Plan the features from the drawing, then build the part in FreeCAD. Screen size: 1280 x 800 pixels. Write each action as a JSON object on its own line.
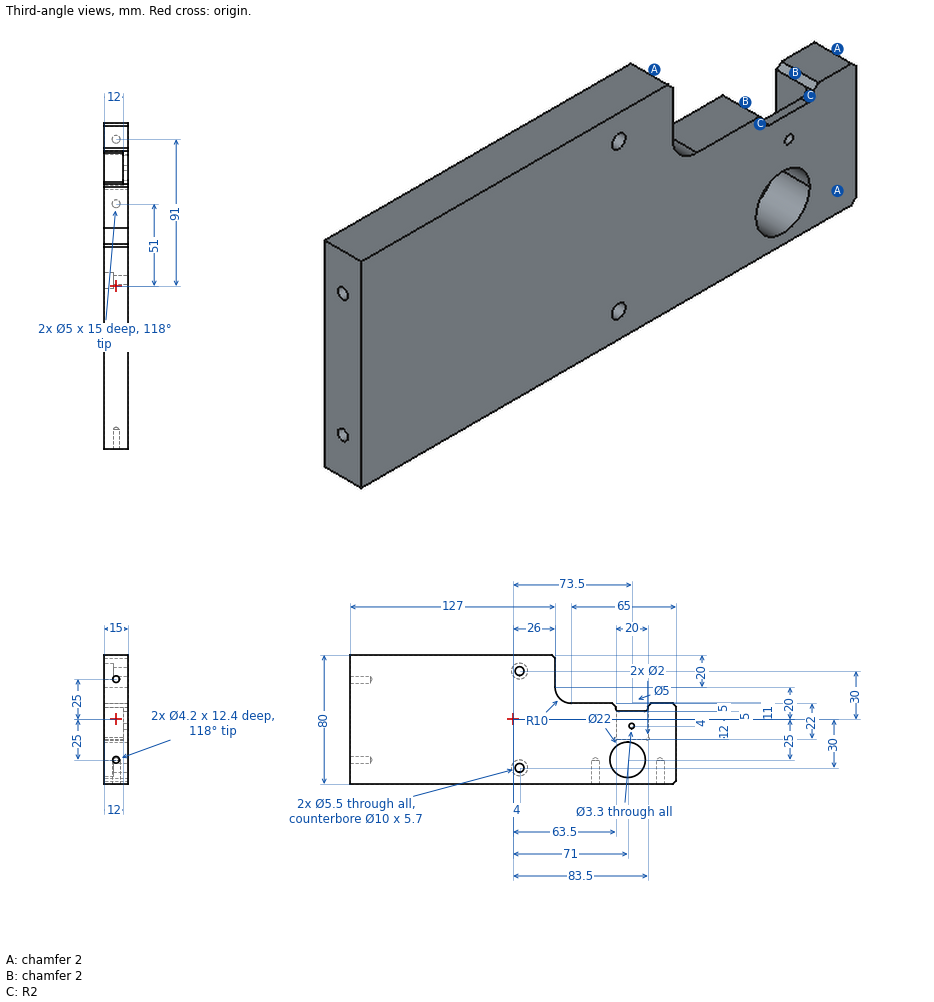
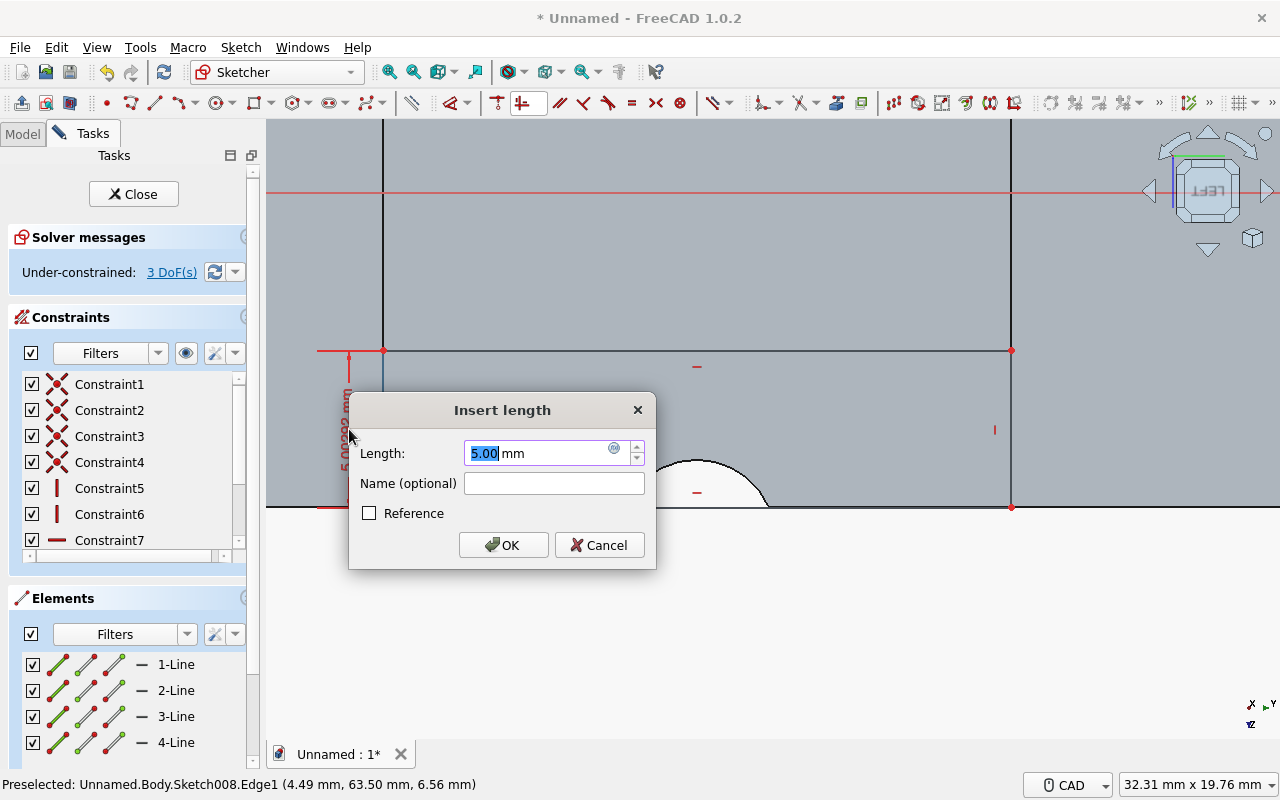
{"action": "type", "text": "5"}
{"action": "key", "text": "Return"}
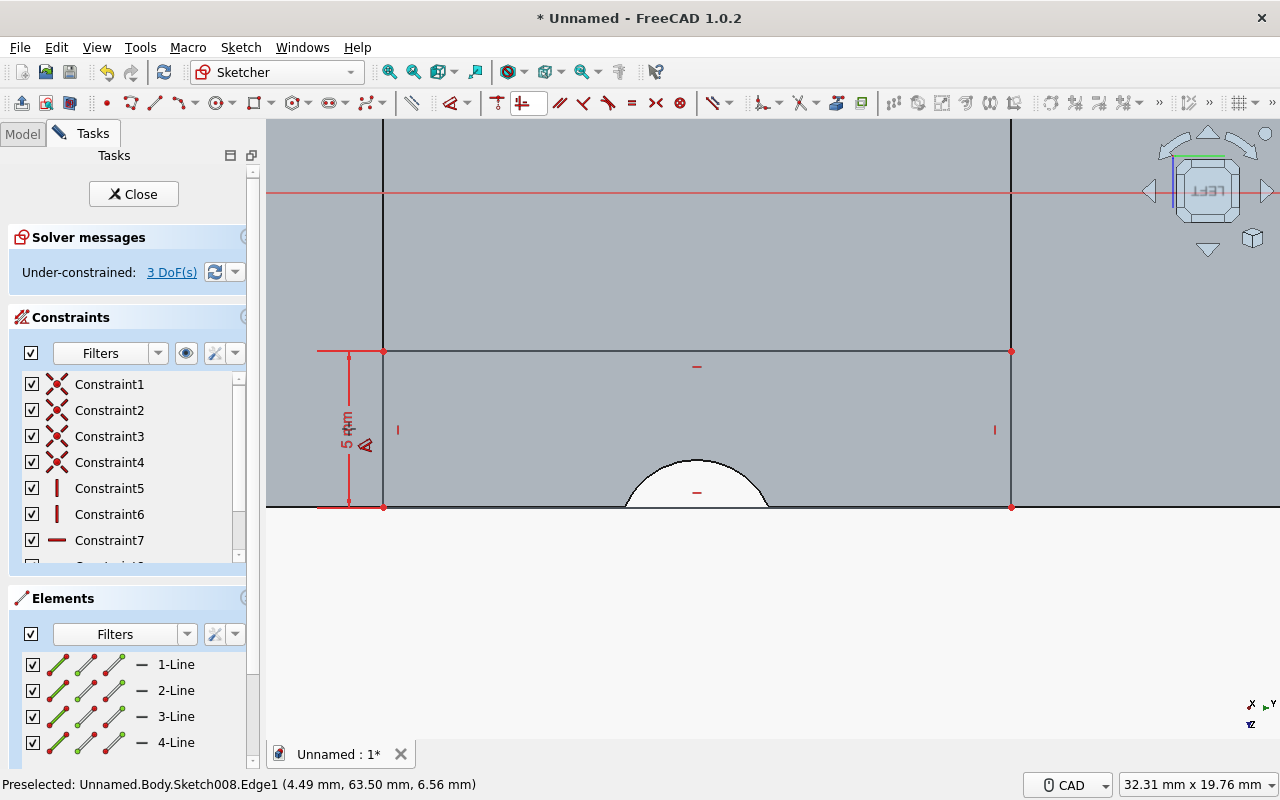
{"action": "left_click", "coordinate": [571, 508]}
{"action": "left_click", "coordinate": [697, 542]}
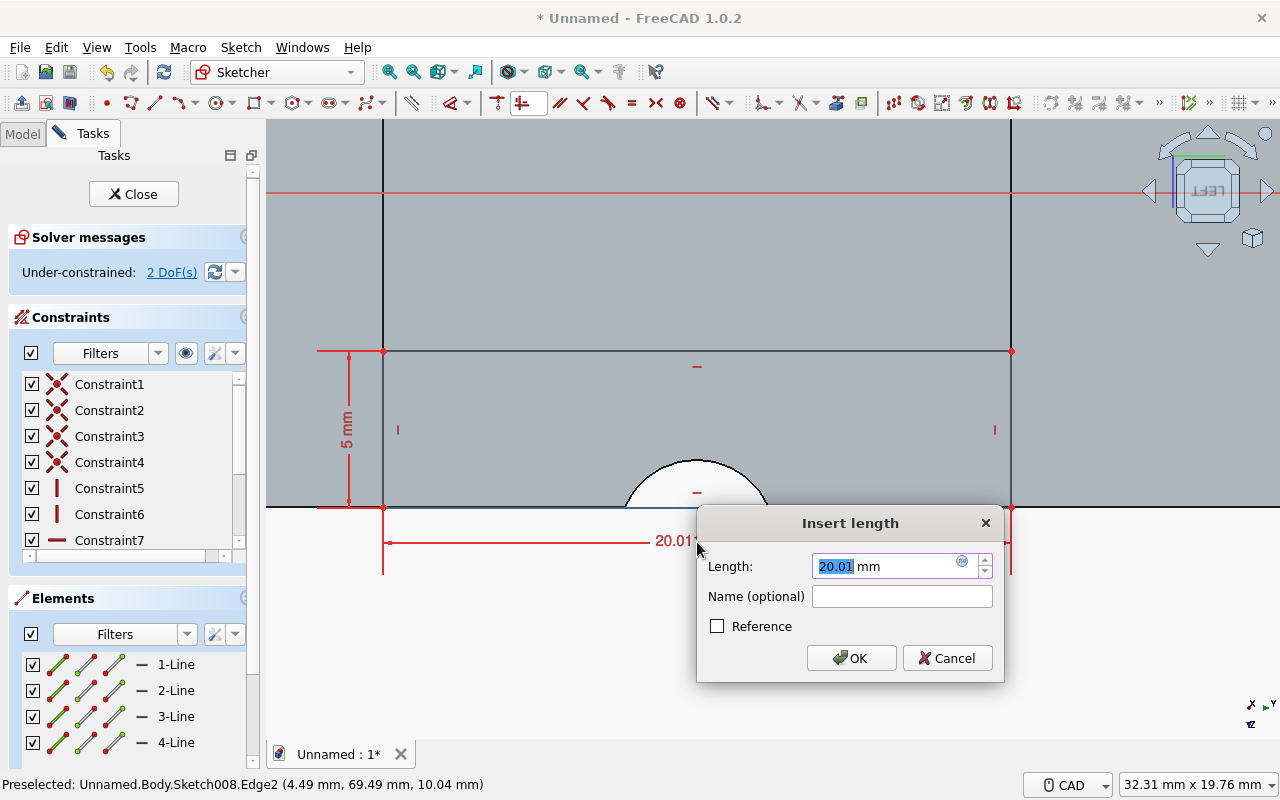
{"action": "type", "text": "20"}
{"action": "key", "text": "Return"}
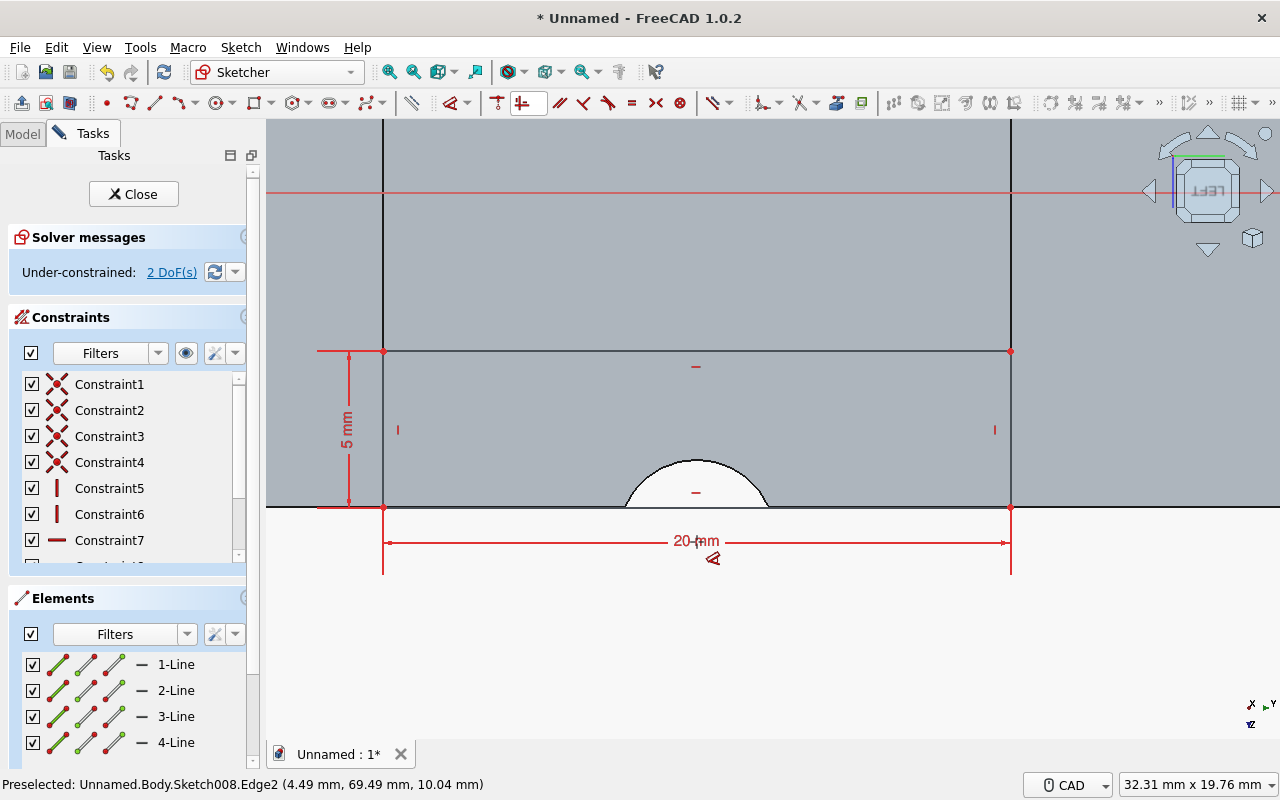
{"action": "left_click", "coordinate": [383, 351]}
{"action": "left_click", "coordinate": [417, 272]}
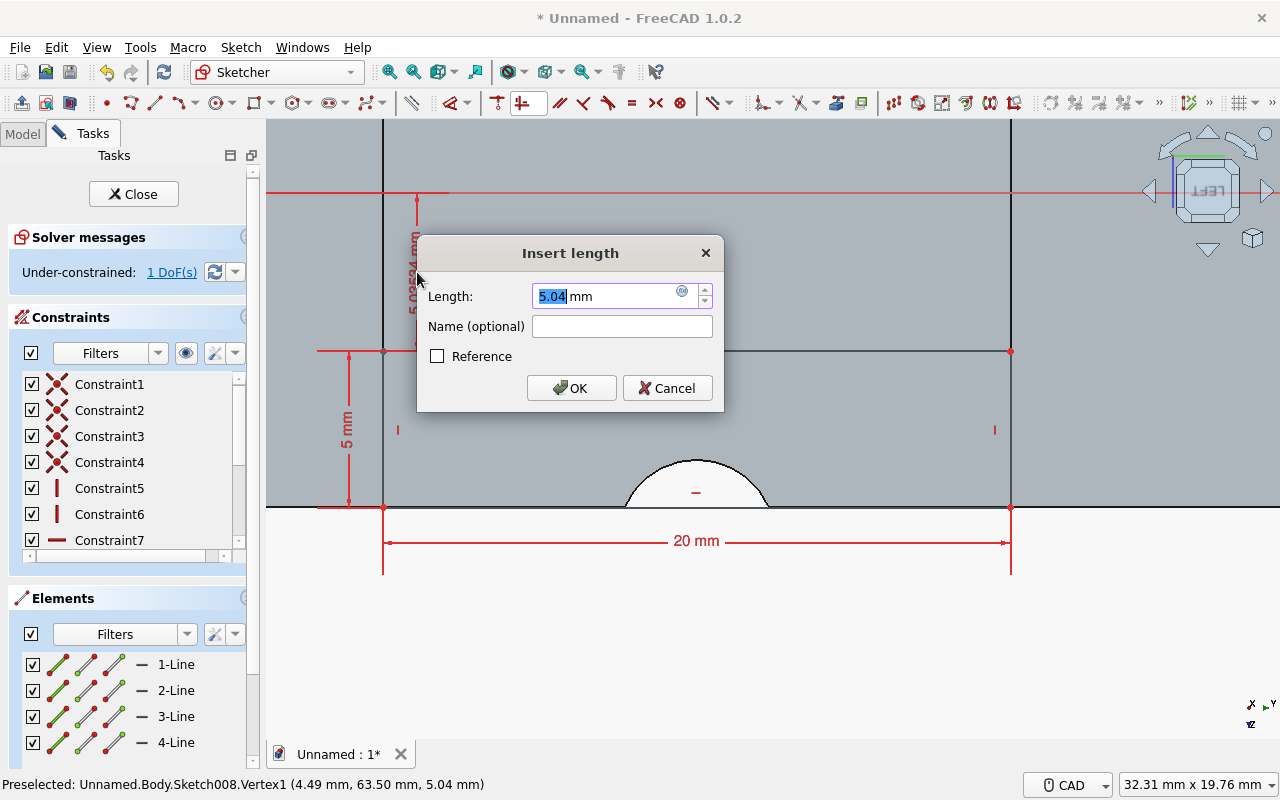
{"action": "type", "text": "5"}
{"action": "key", "text": "Return"}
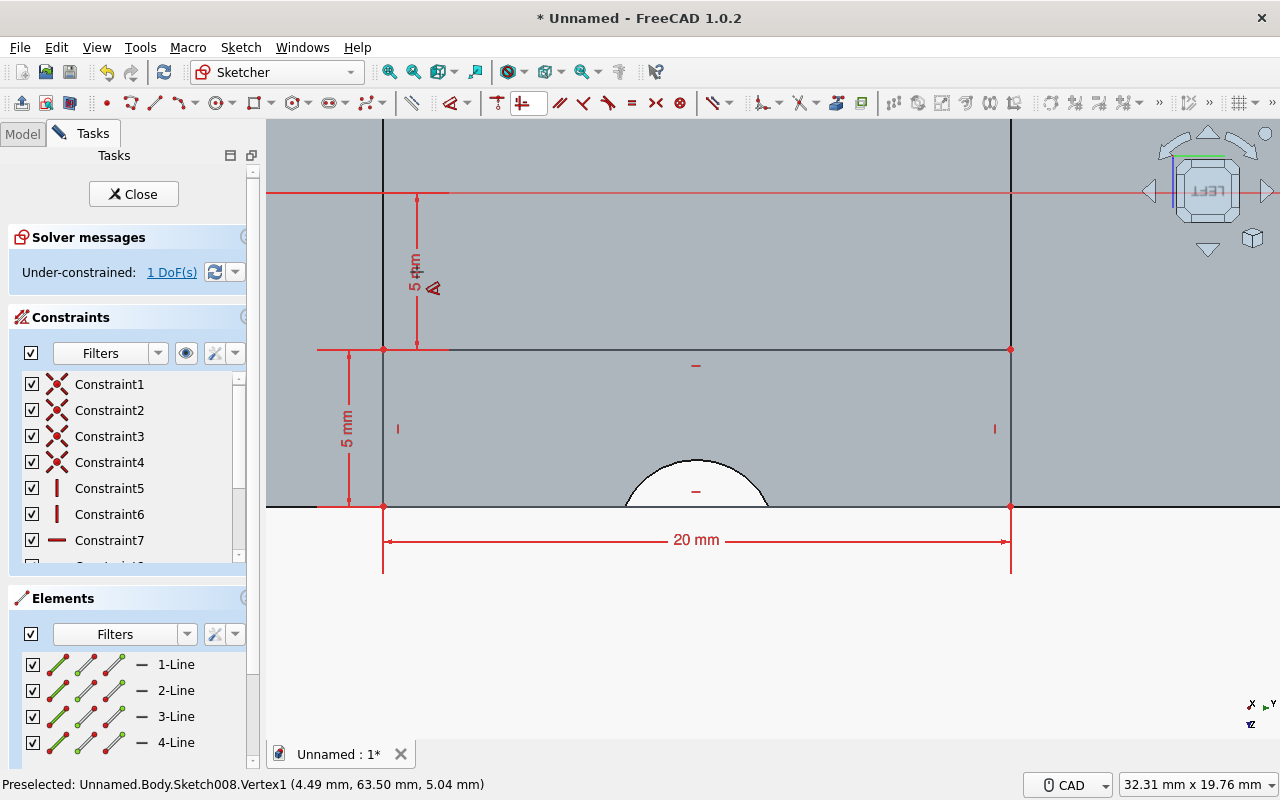
{"action": "left_click", "coordinate": [383, 350]}
{"action": "left_click", "coordinate": [339, 159]}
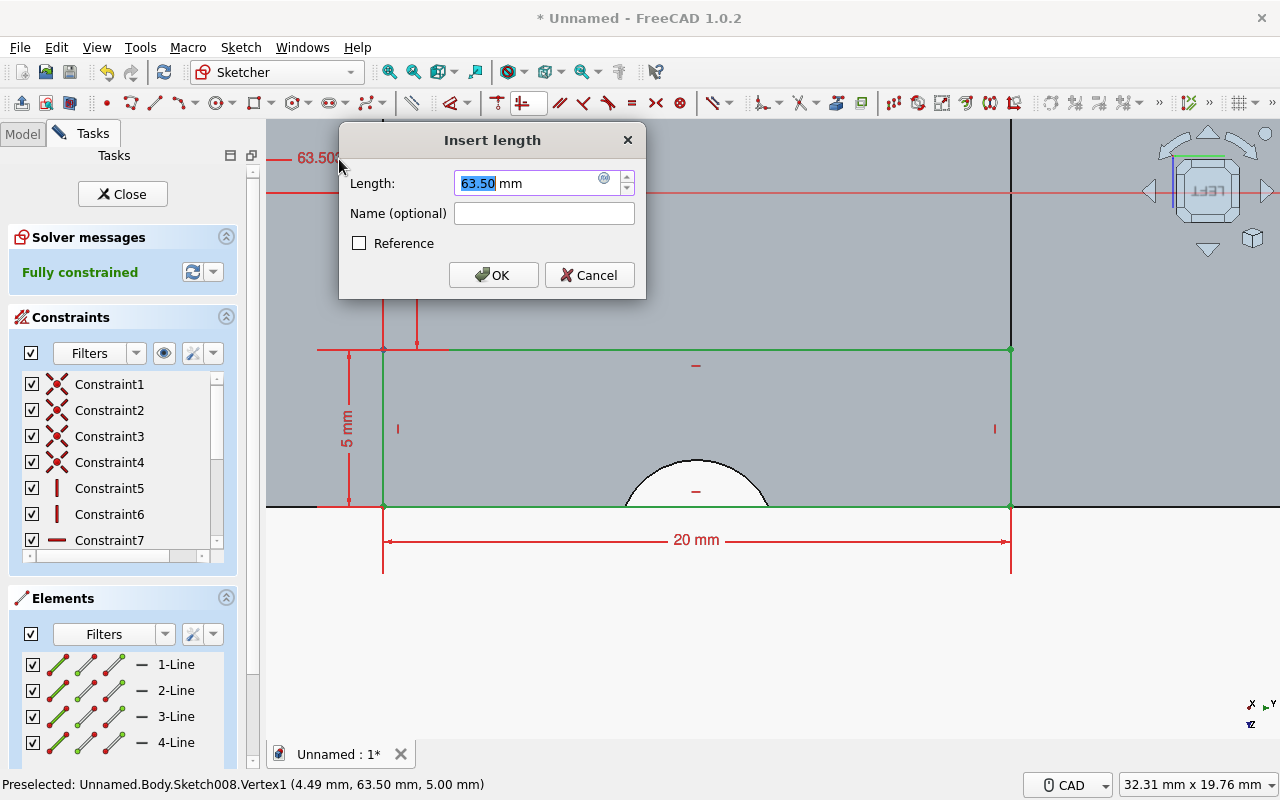
{"action": "type", "text": "63.5"}
{"action": "key", "text": "Return"}
{"action": "key", "text": "Escape"}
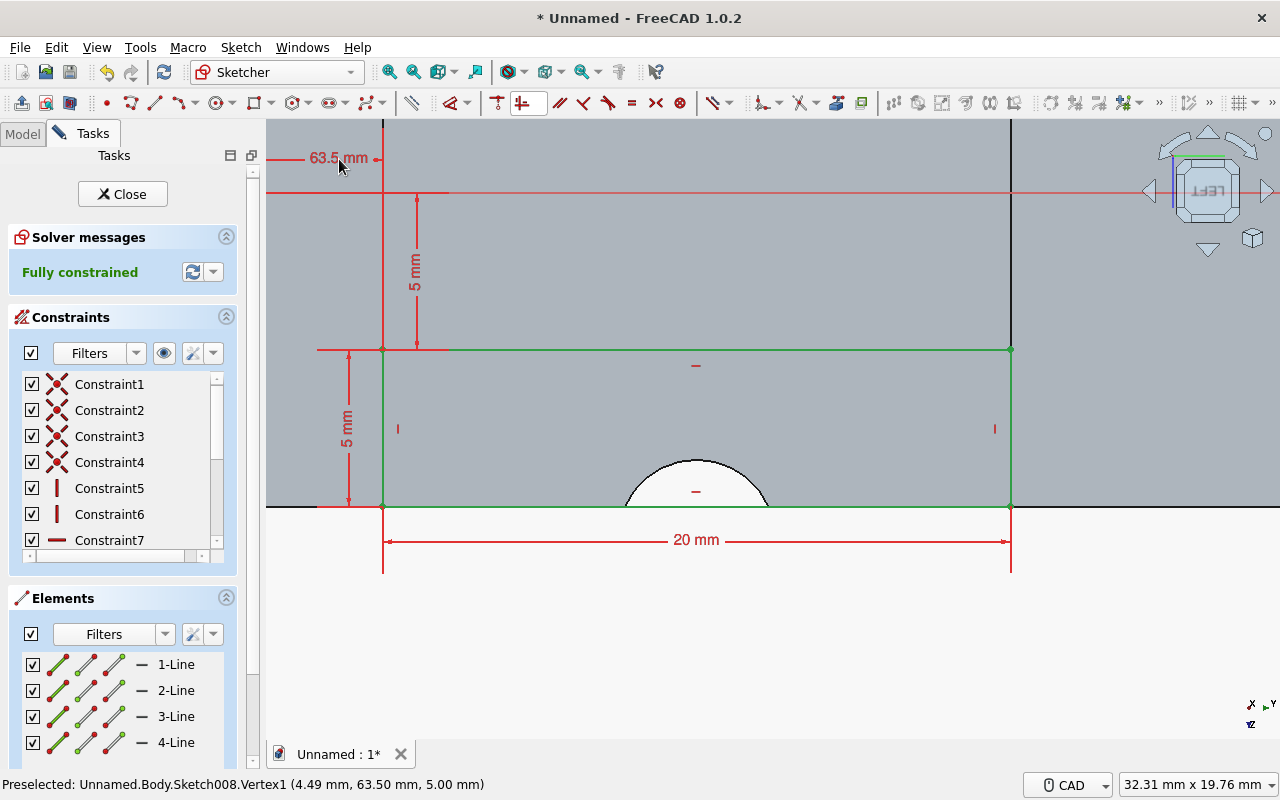
{"action": "left_click", "coordinate": [123, 194]}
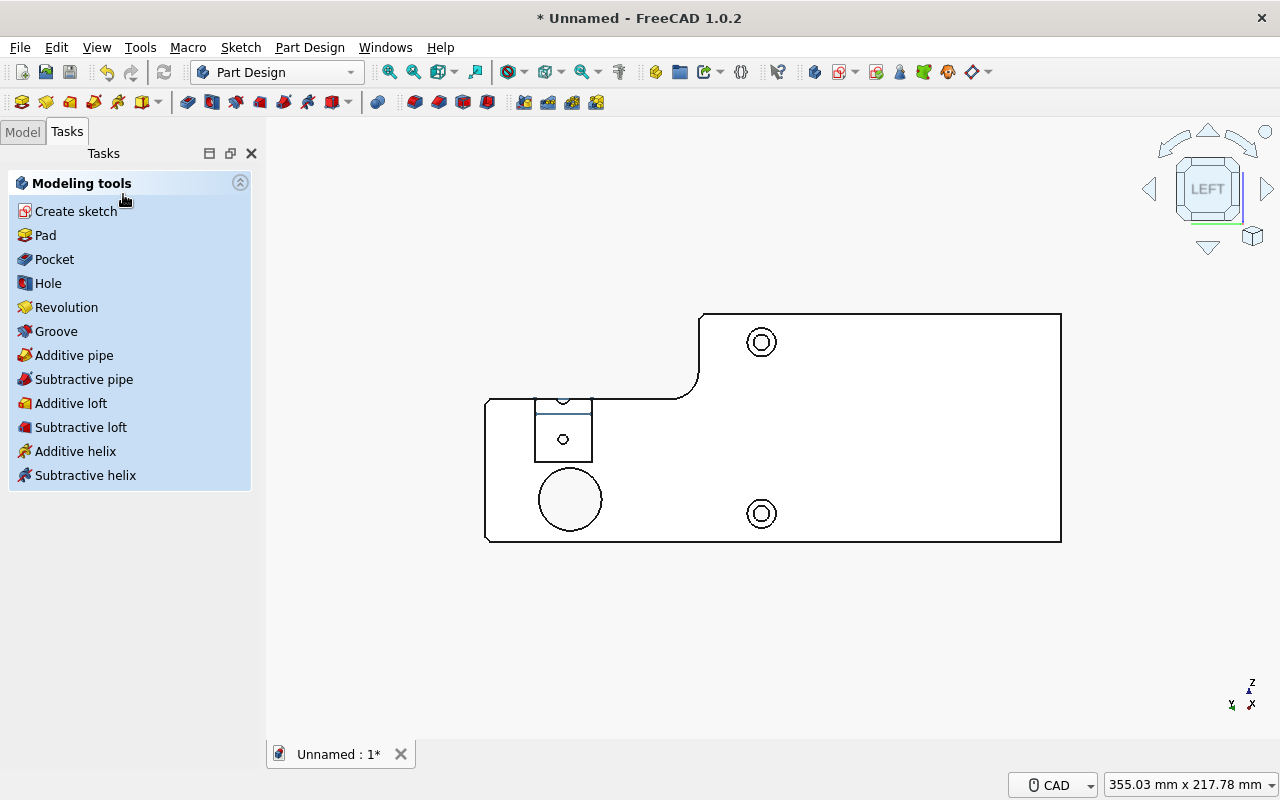
{"action": "left_click", "coordinate": [188, 102]}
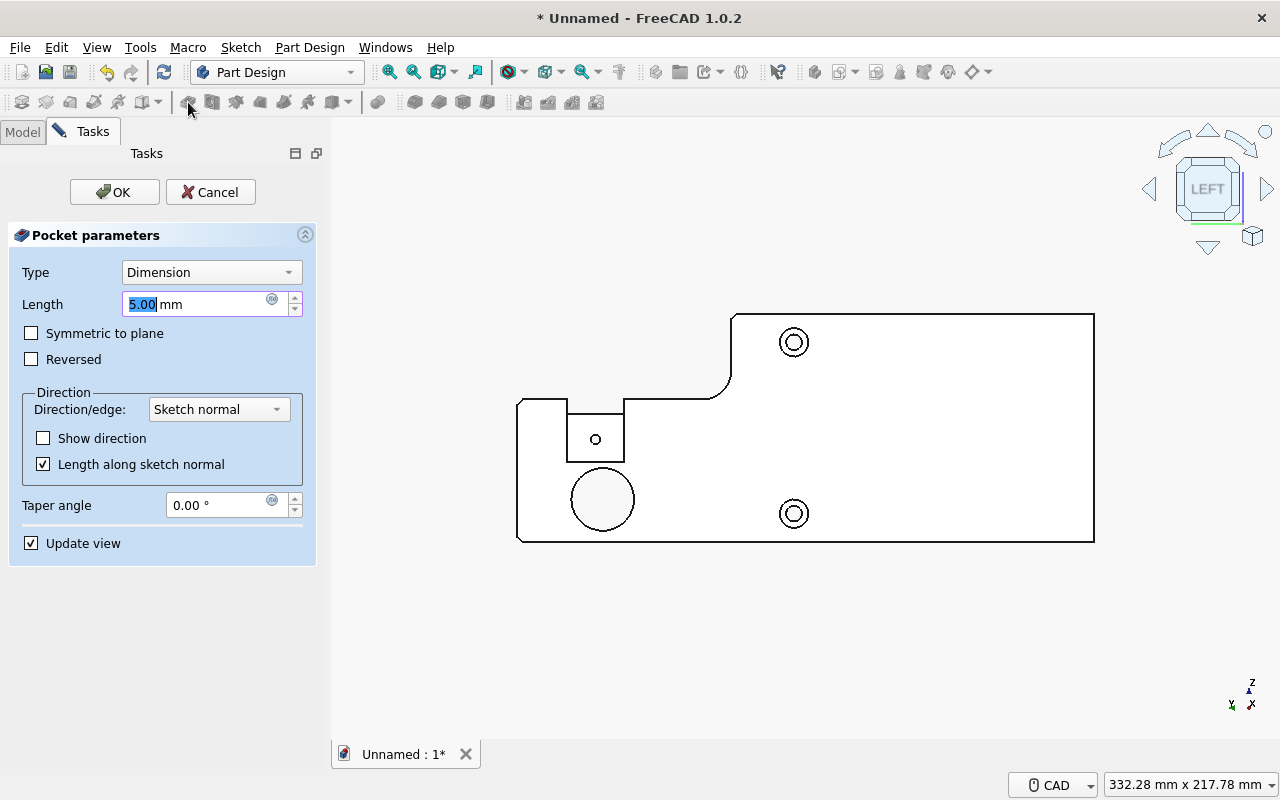
{"action": "left_click", "coordinate": [212, 272]}